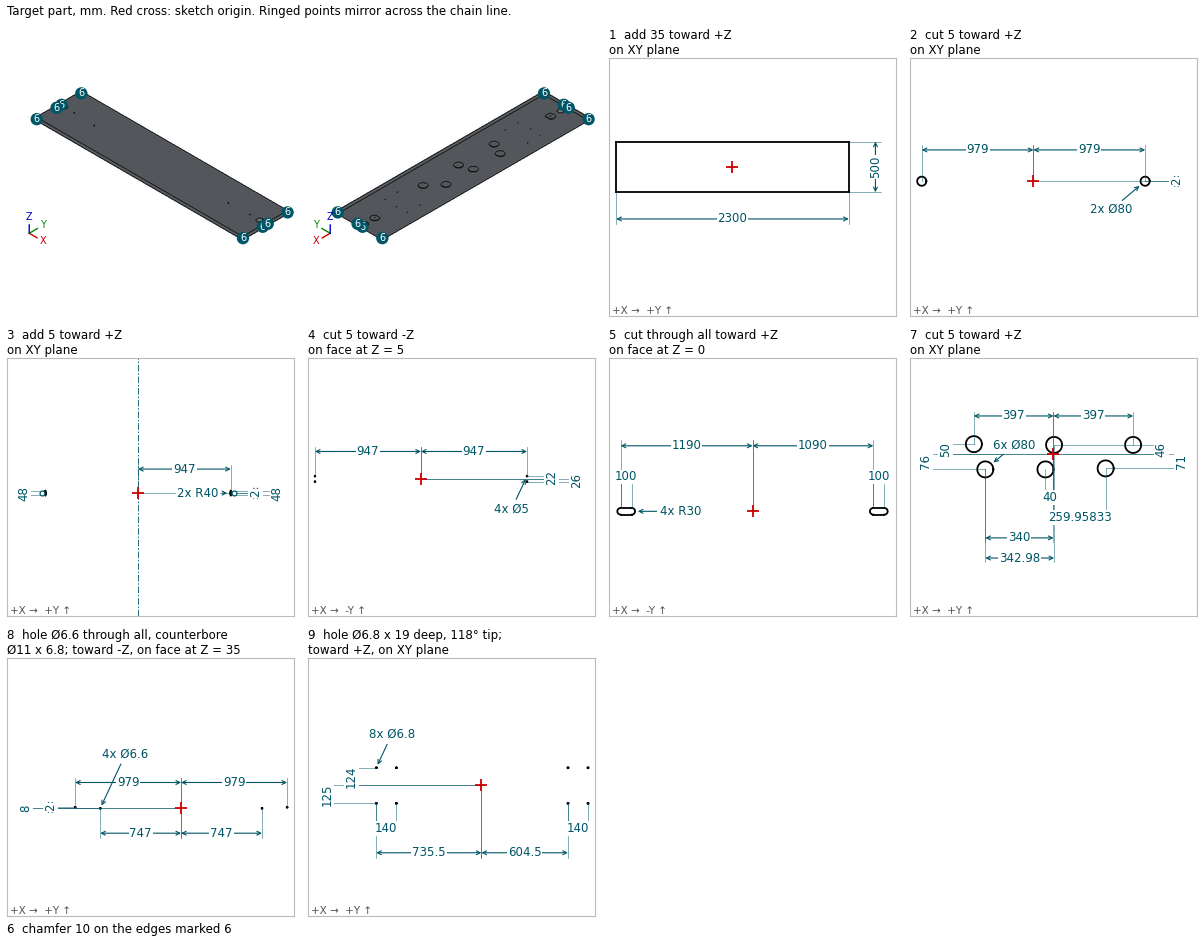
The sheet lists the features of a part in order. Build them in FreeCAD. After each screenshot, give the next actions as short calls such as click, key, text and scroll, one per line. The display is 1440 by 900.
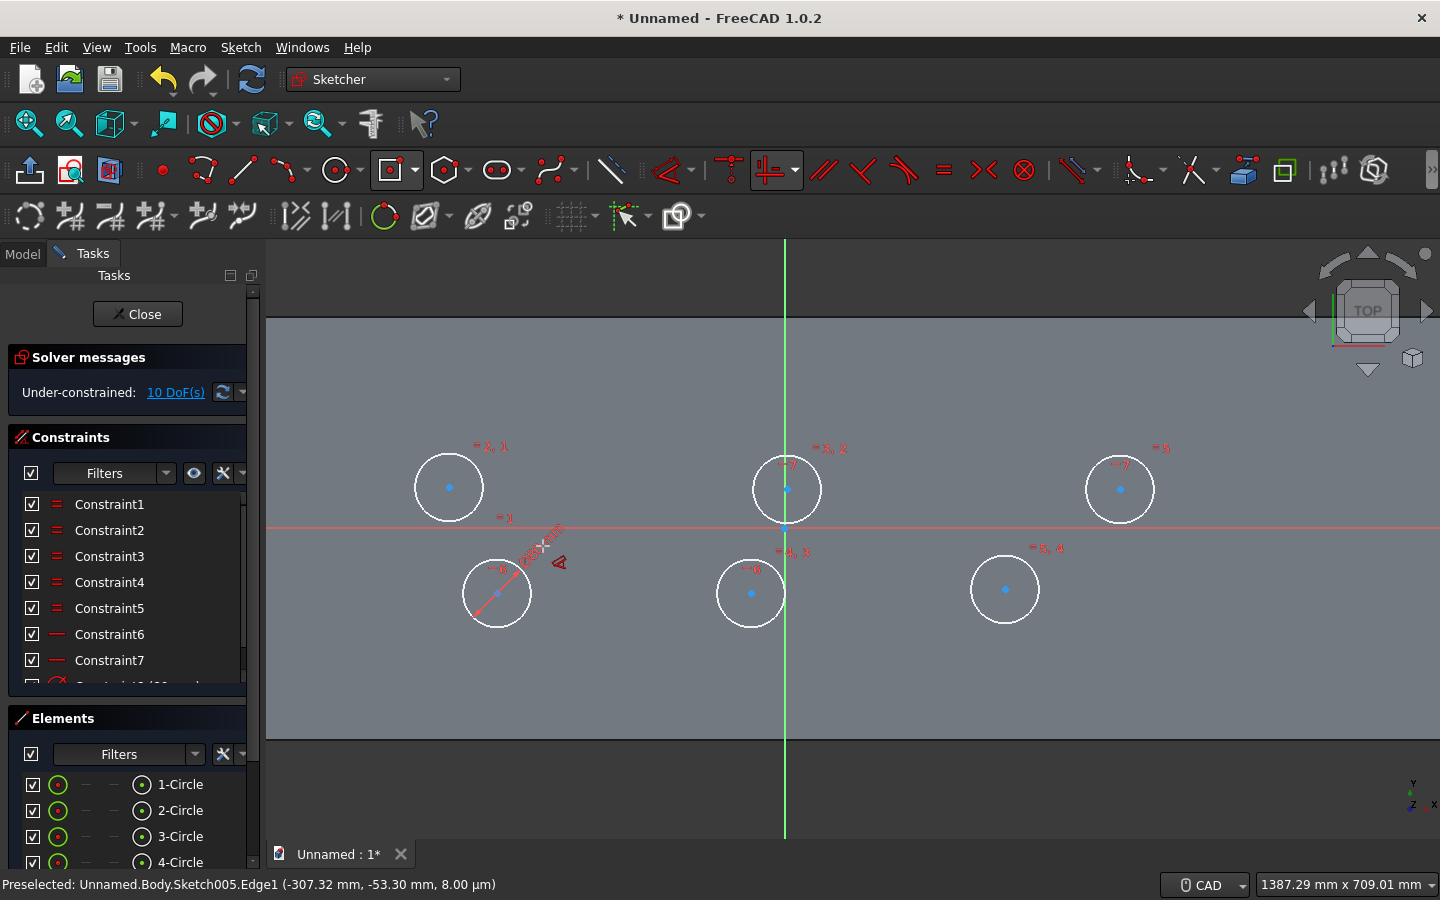
click(497, 593)
click(463, 561)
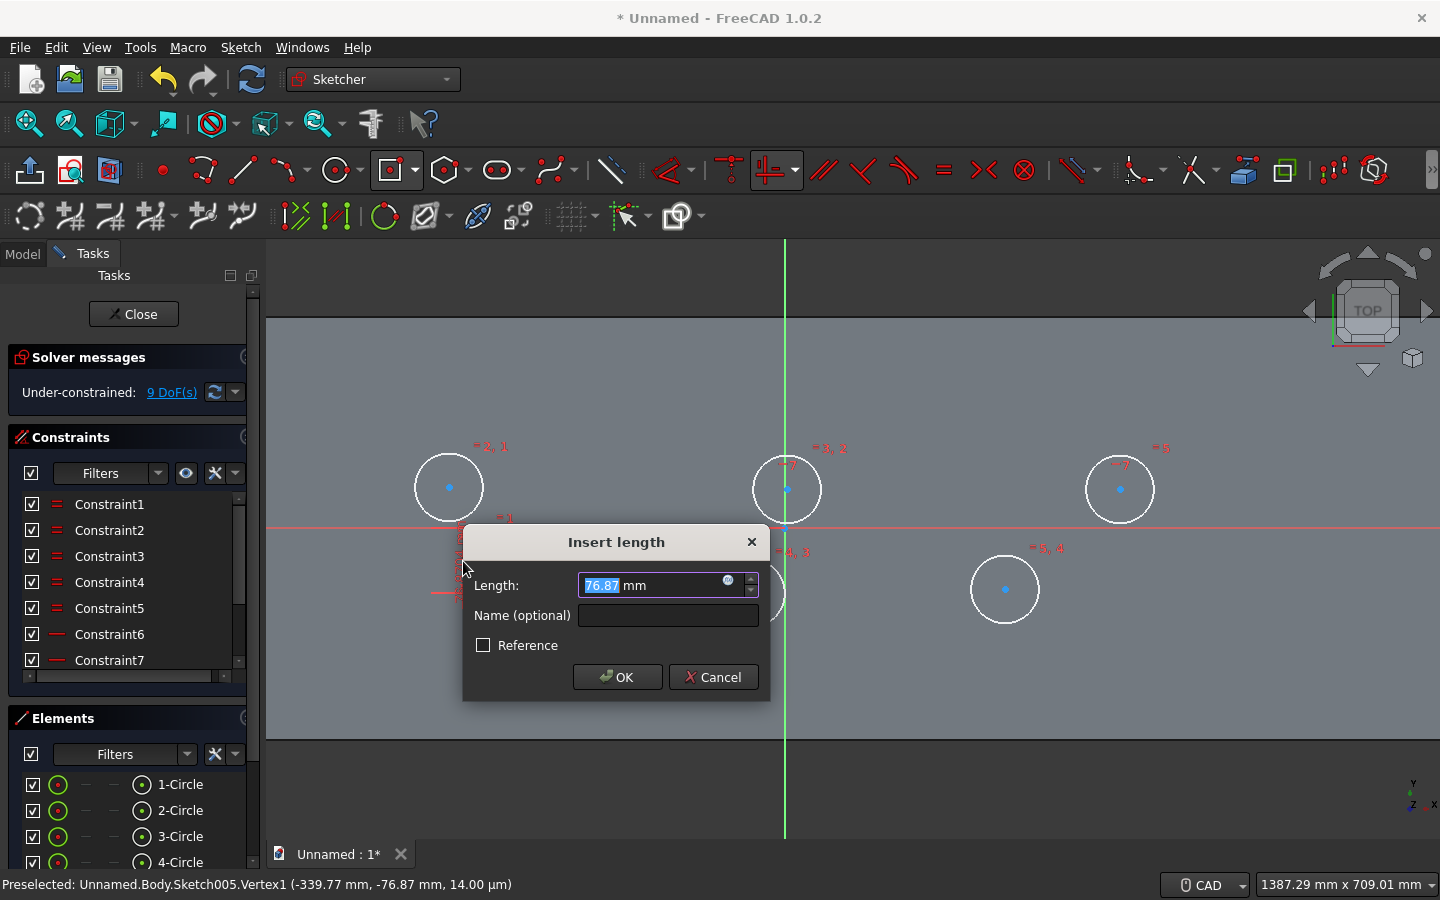
text(76)
key(Return)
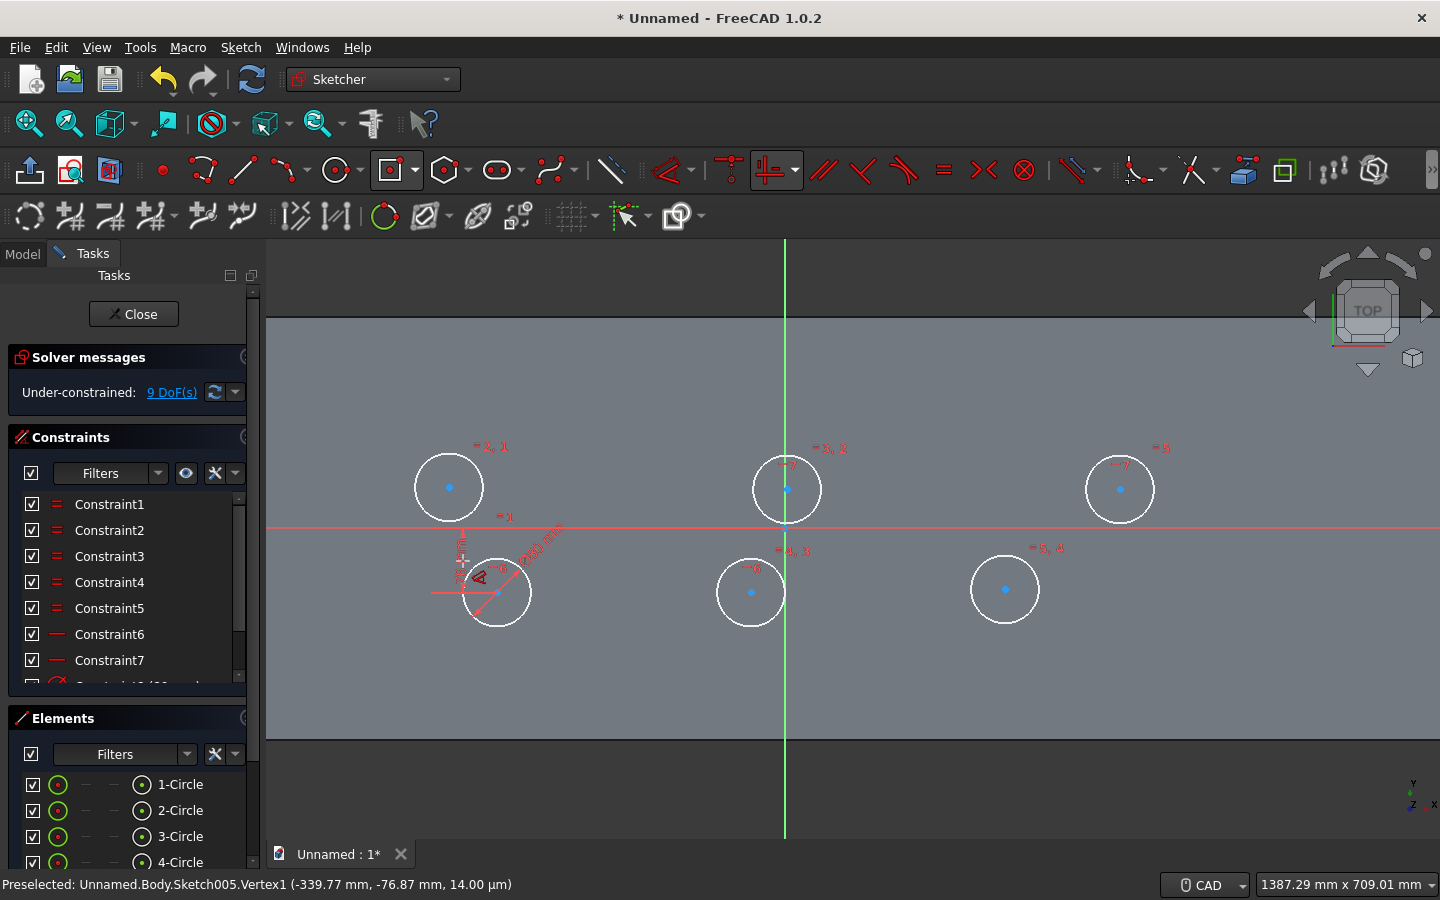
click(449, 487)
click(391, 508)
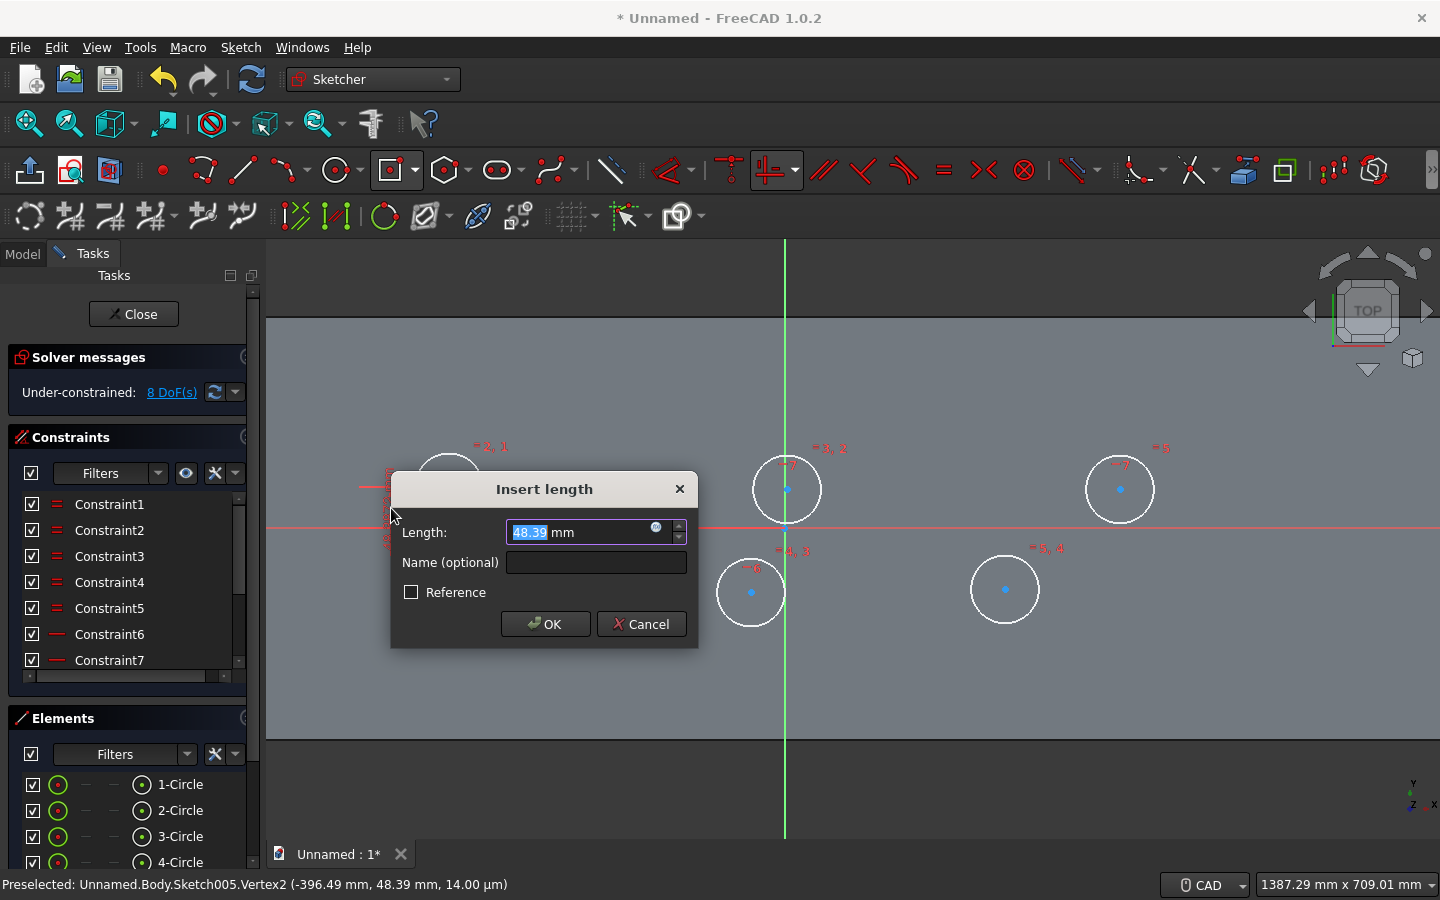
text(50)
key(Return)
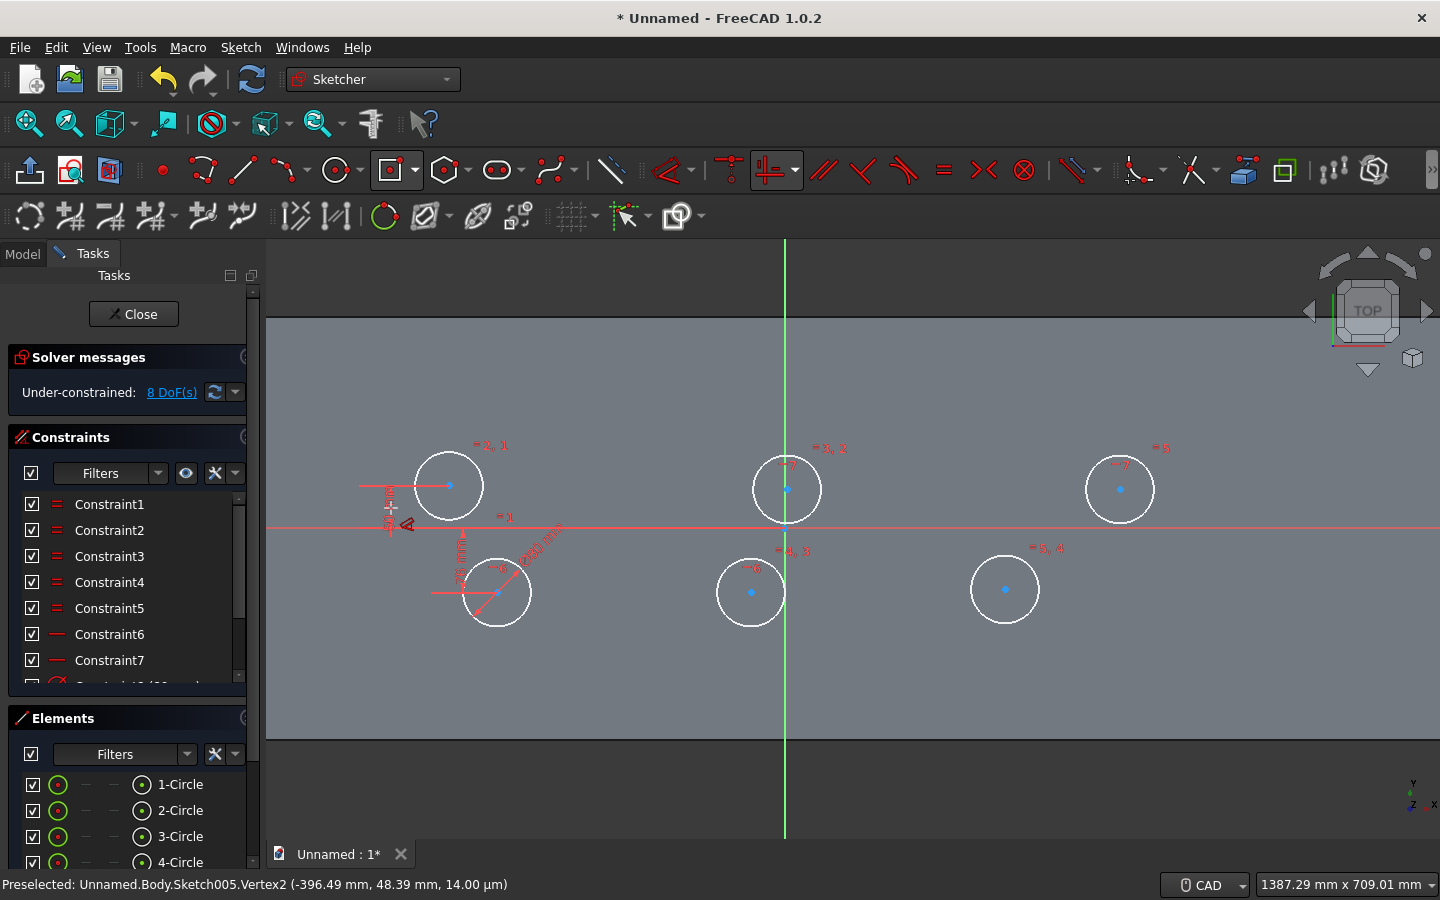
click(787, 489)
click(845, 509)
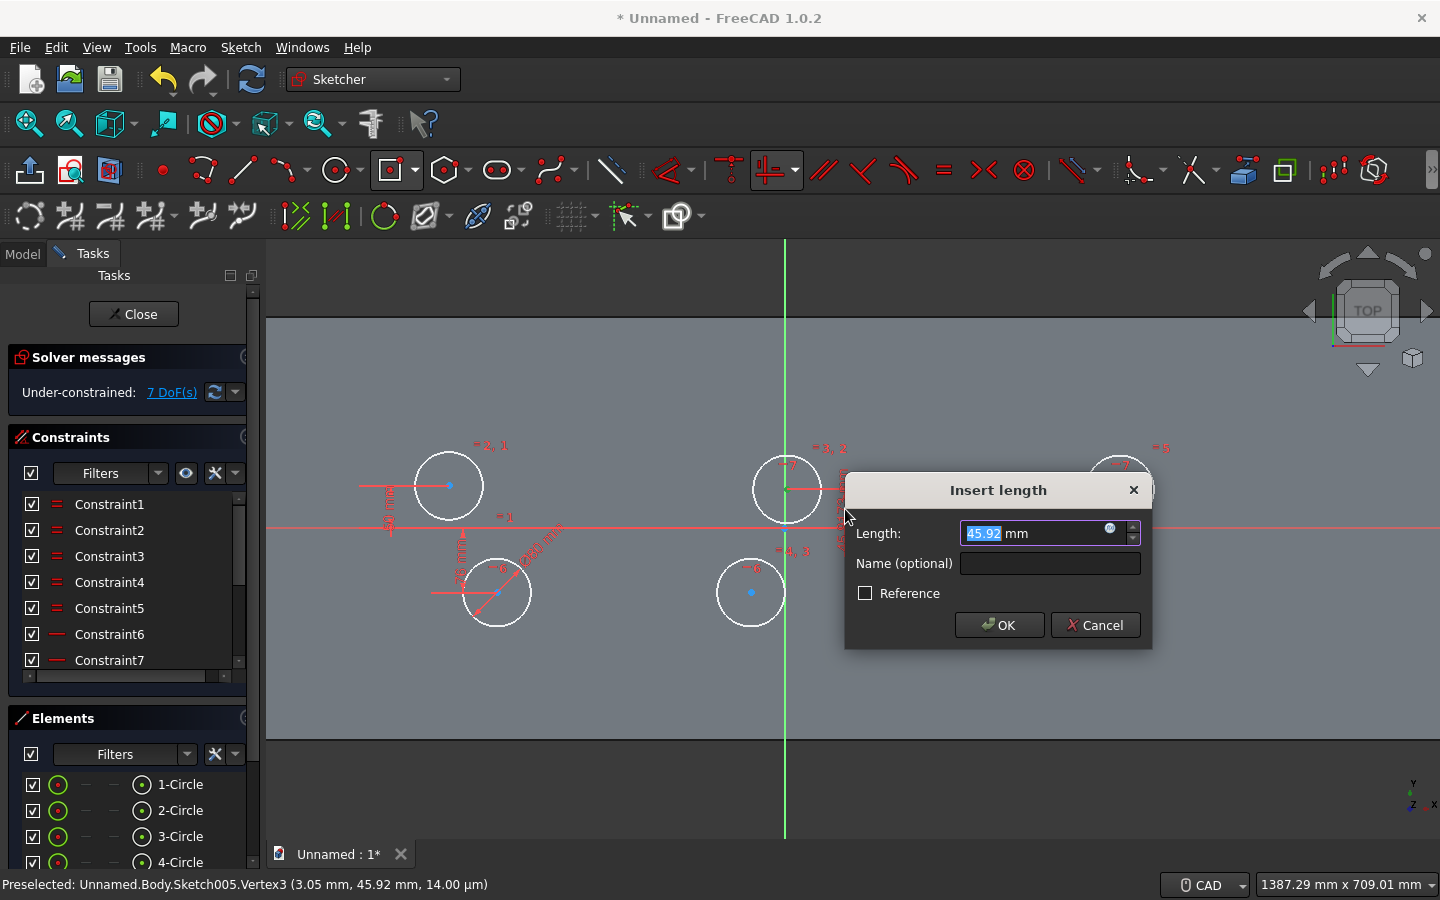
text(46)
key(Return)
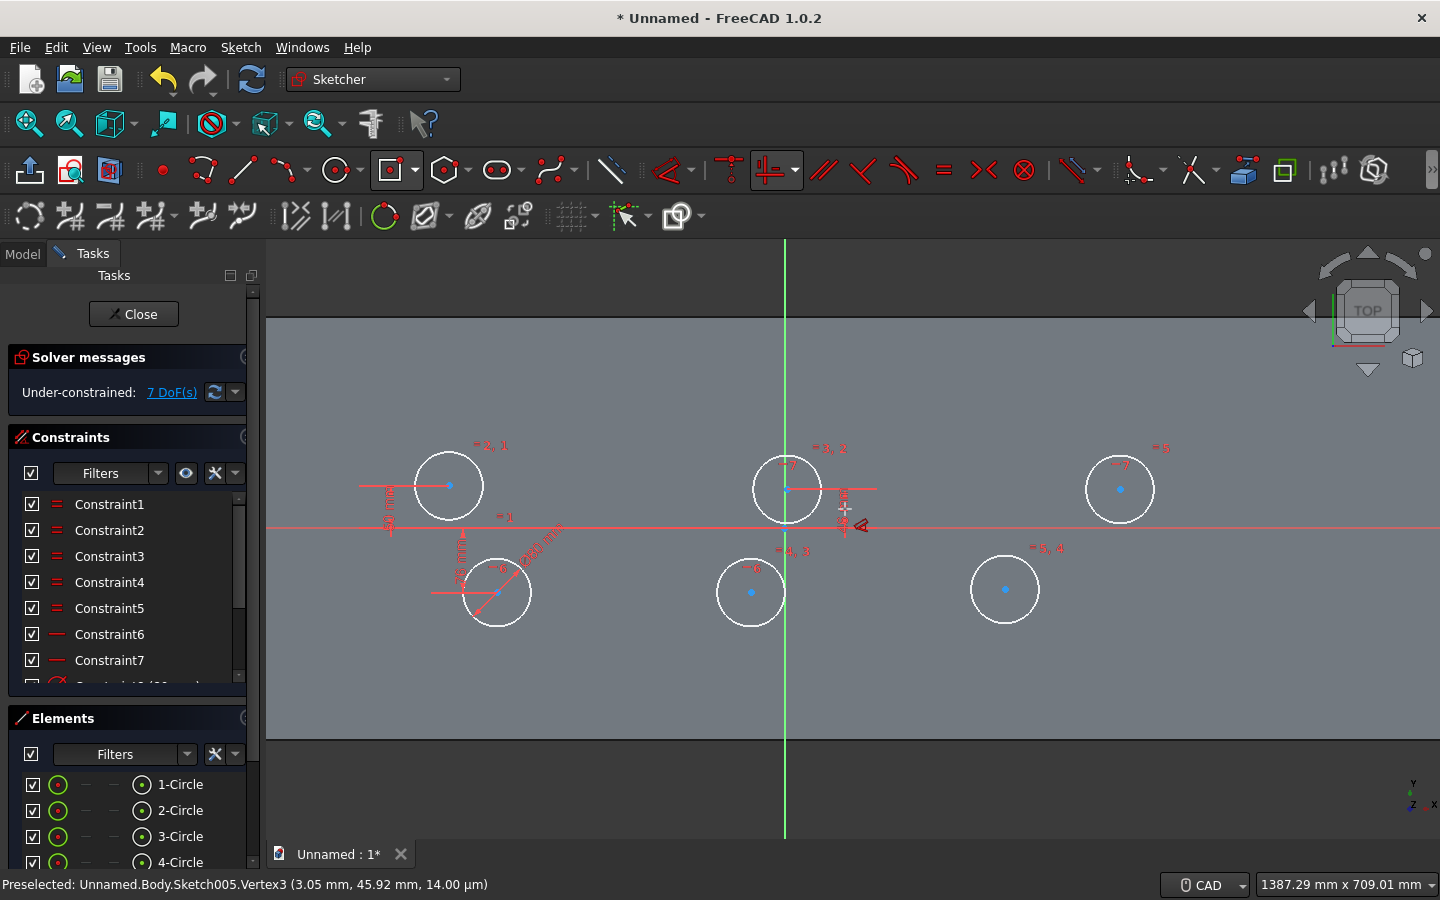
click(751, 593)
click(768, 494)